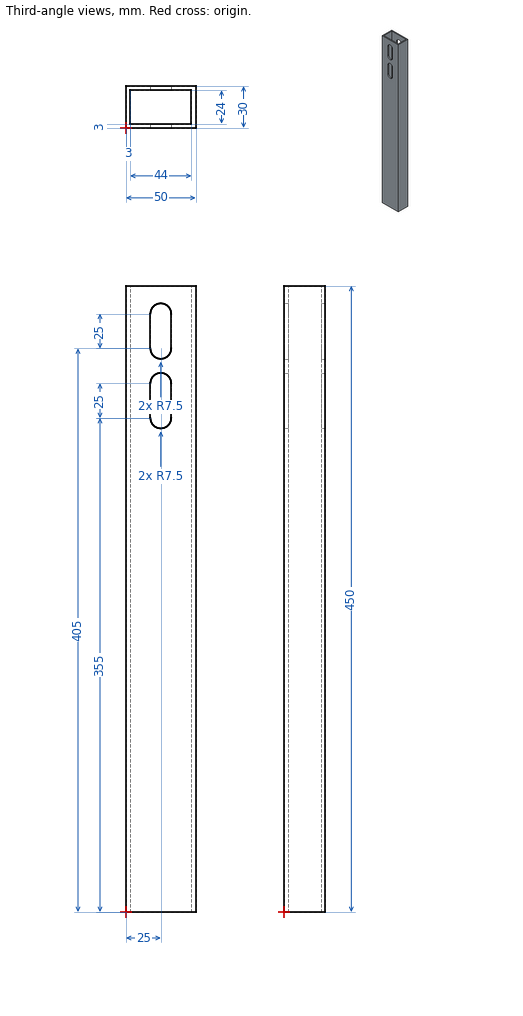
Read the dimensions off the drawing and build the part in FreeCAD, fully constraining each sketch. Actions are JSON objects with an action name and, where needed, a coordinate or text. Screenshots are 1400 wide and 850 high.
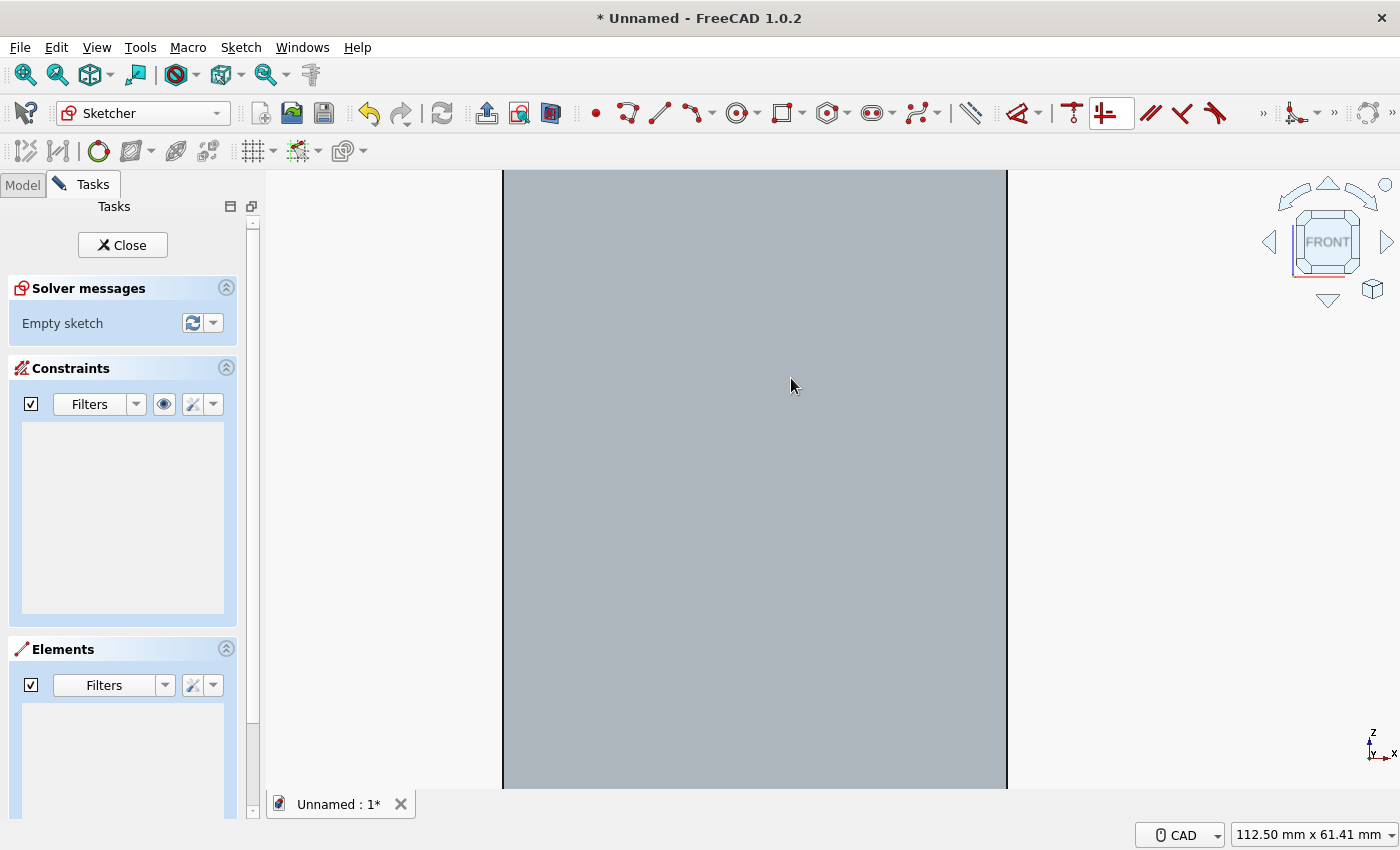
{"action": "left_click", "coordinate": [755, 609]}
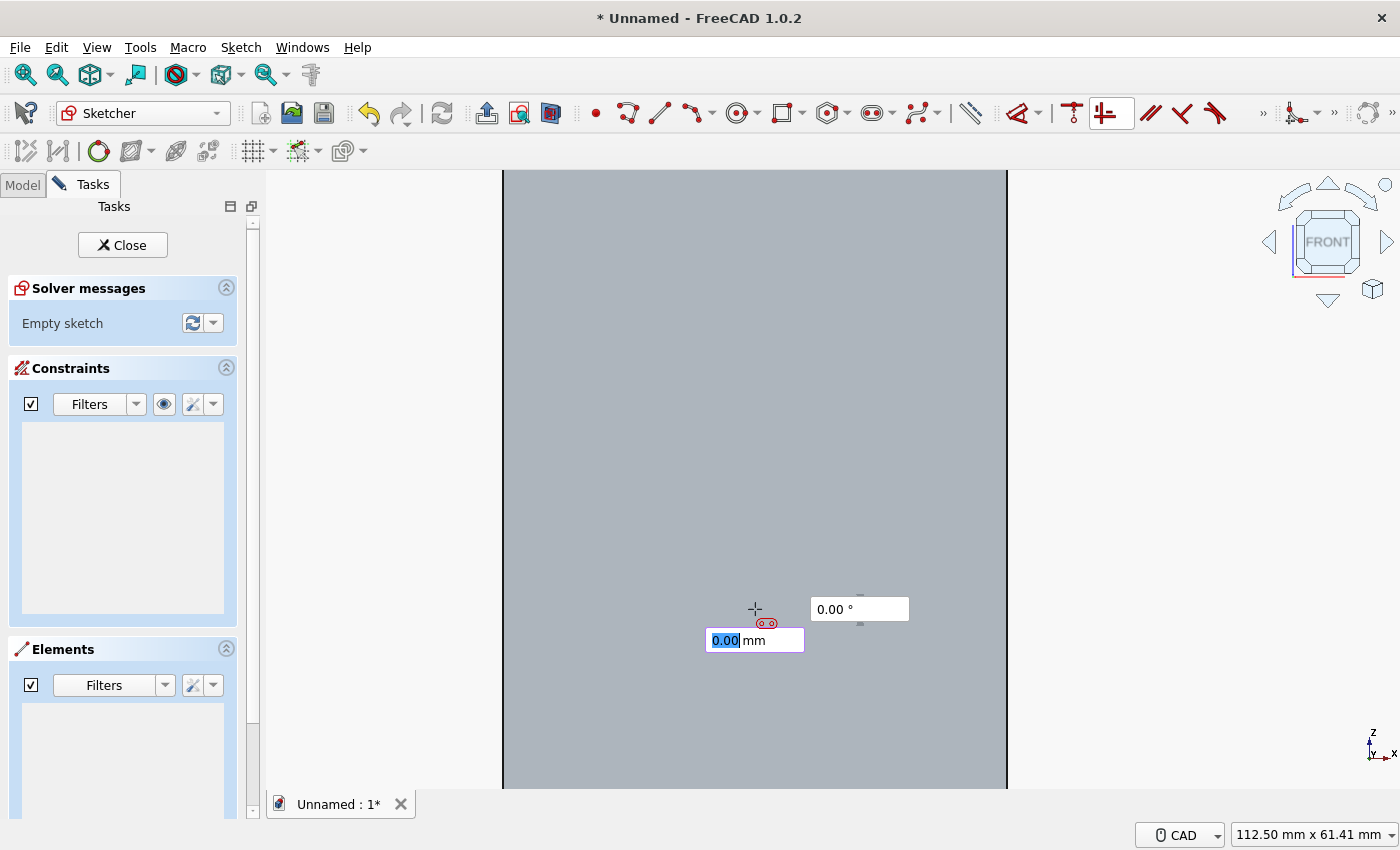
{"action": "left_click", "coordinate": [755, 357]}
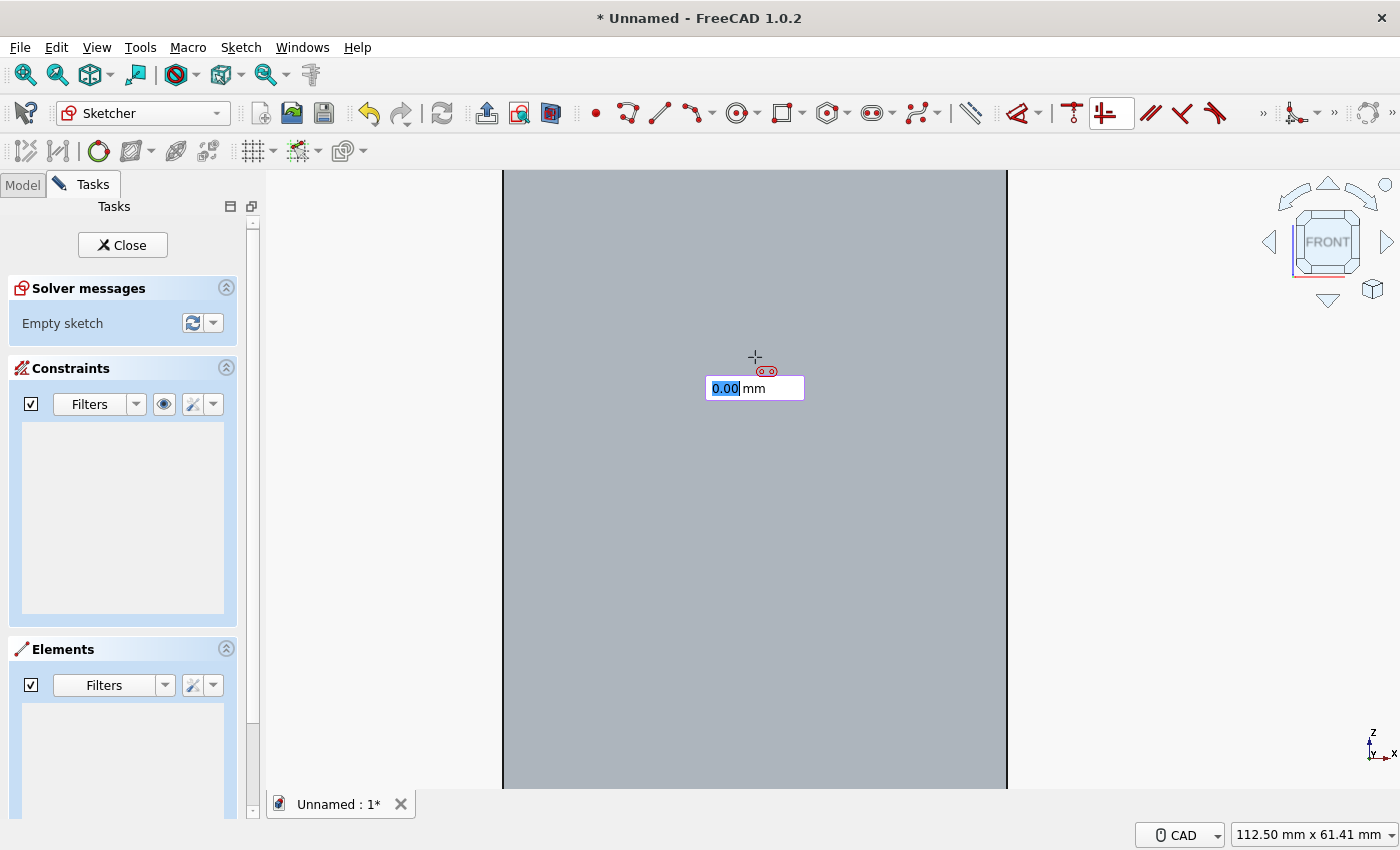
{"action": "left_click", "coordinate": [680, 483]}
{"action": "key", "text": "Escape"}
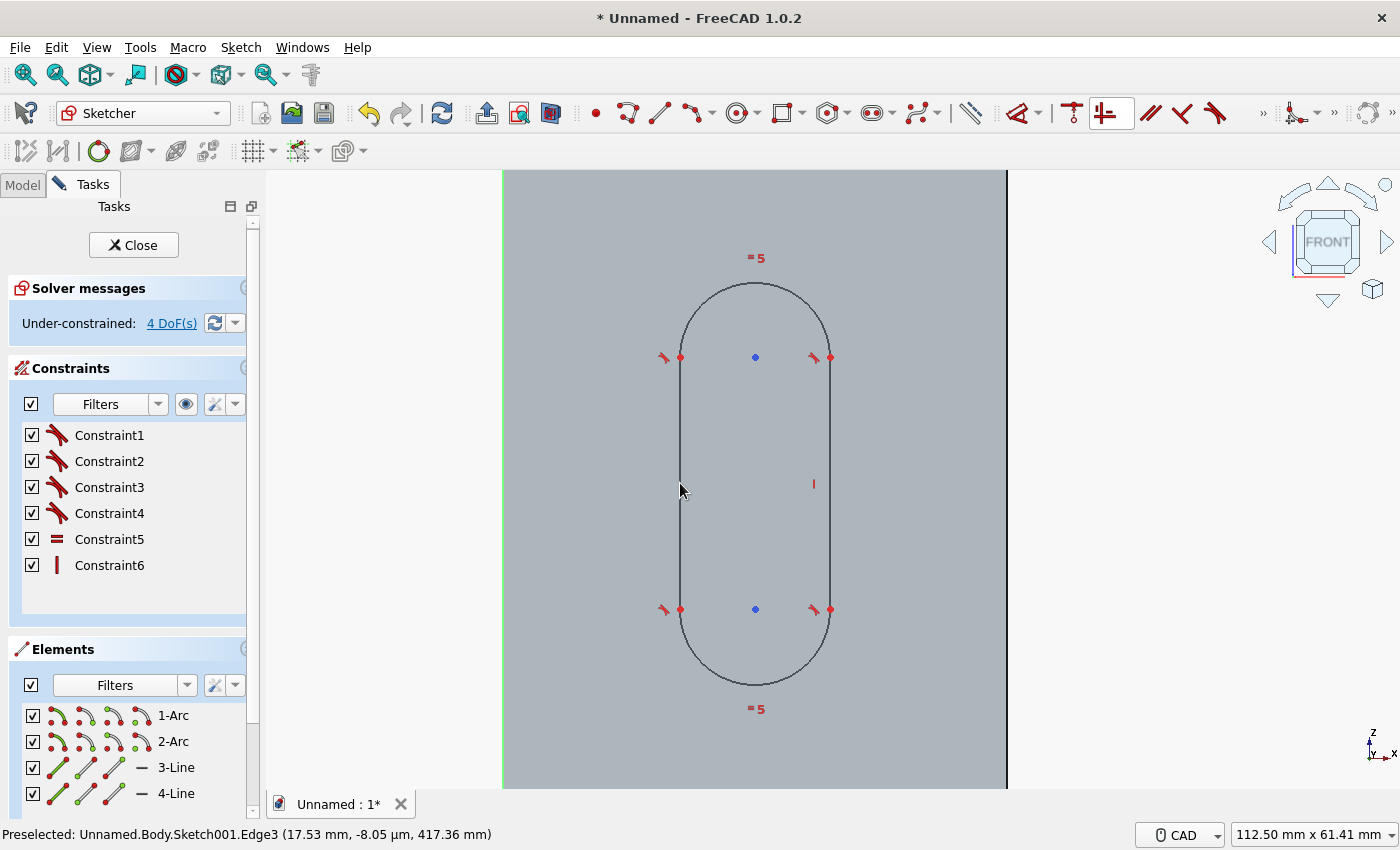
{"action": "left_click", "coordinate": [711, 671]}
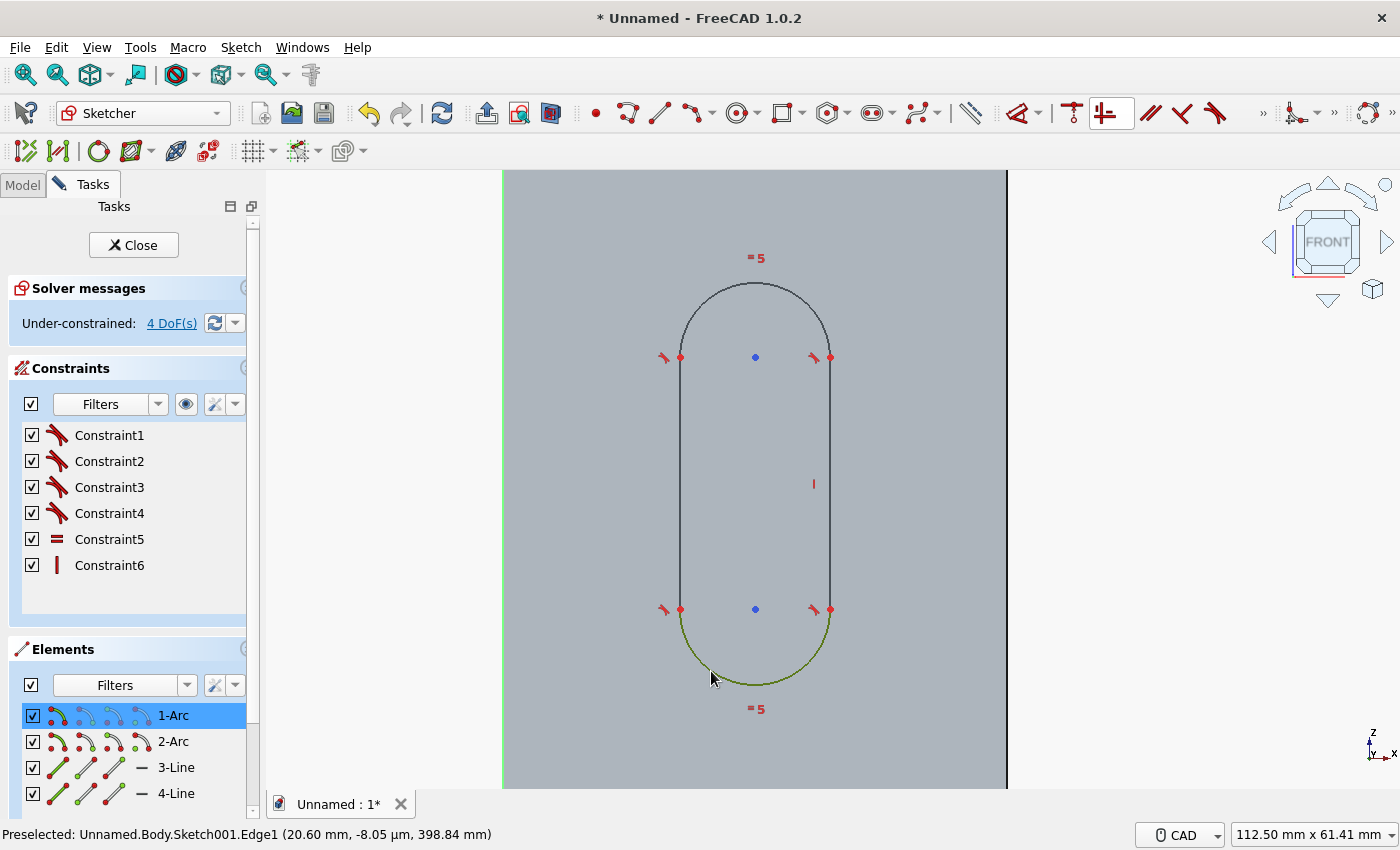
{"action": "key", "text": "k r"}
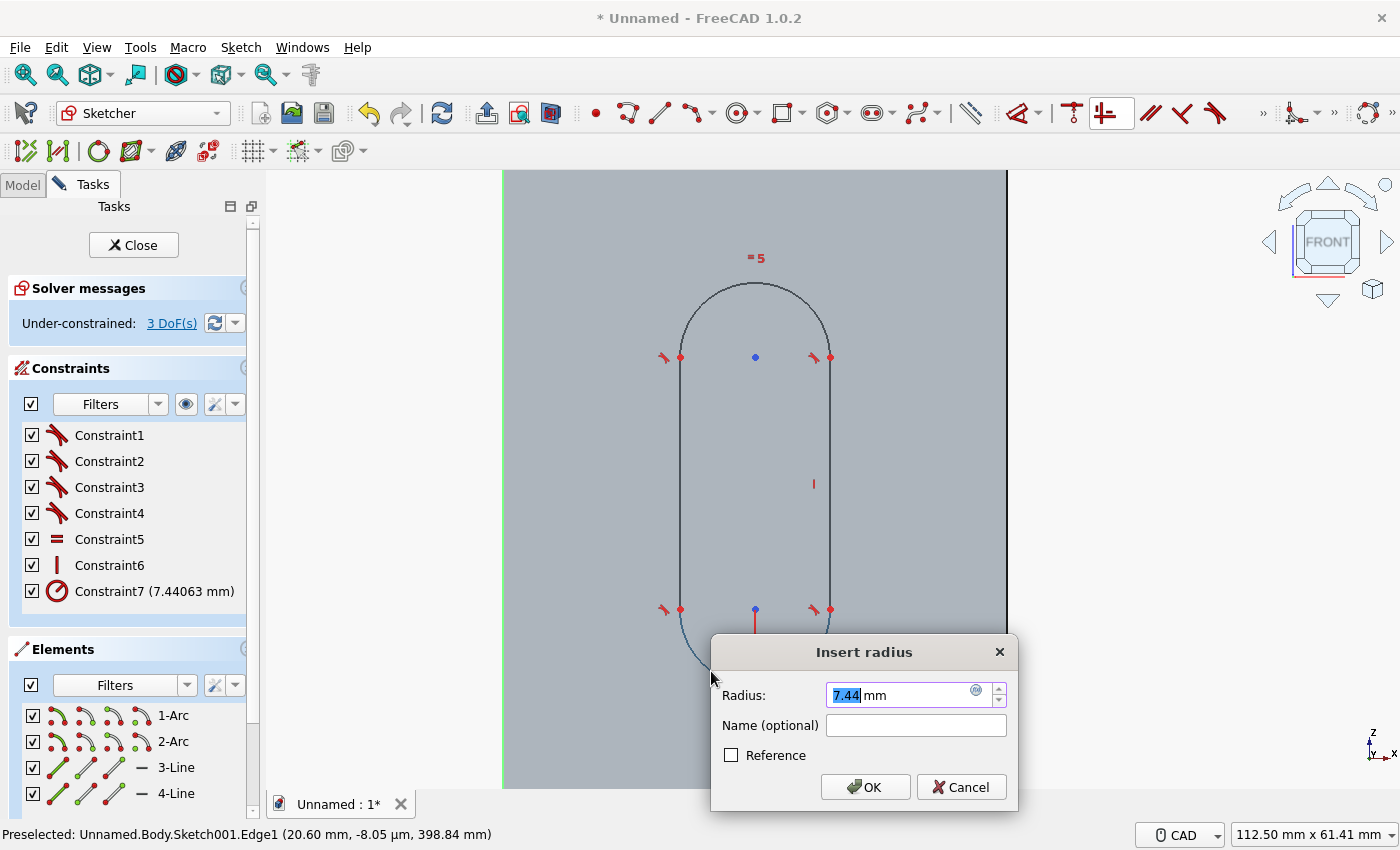
{"action": "type", "text": "7.5"}
{"action": "key", "text": "Return"}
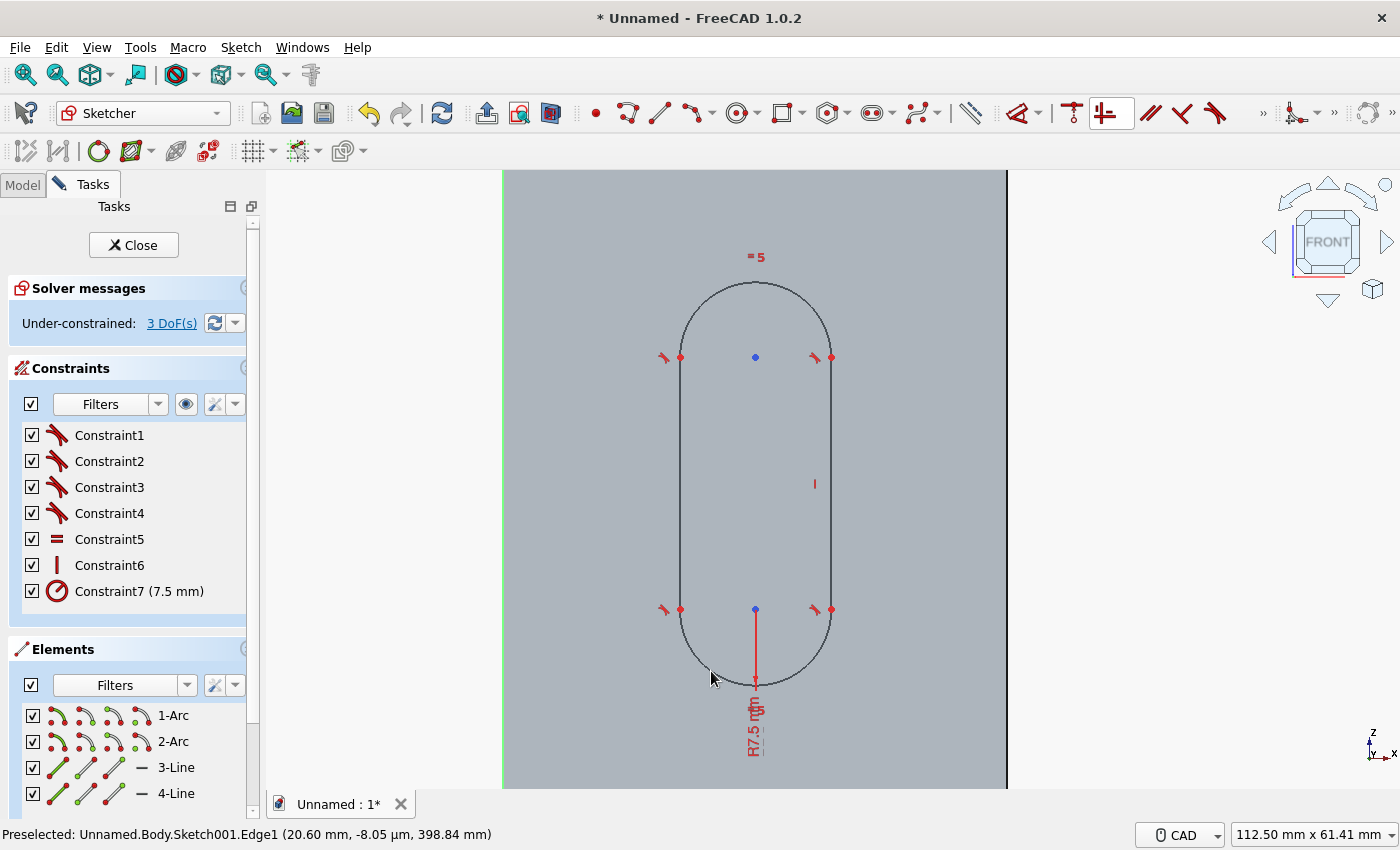
{"action": "left_click", "coordinate": [680, 534]}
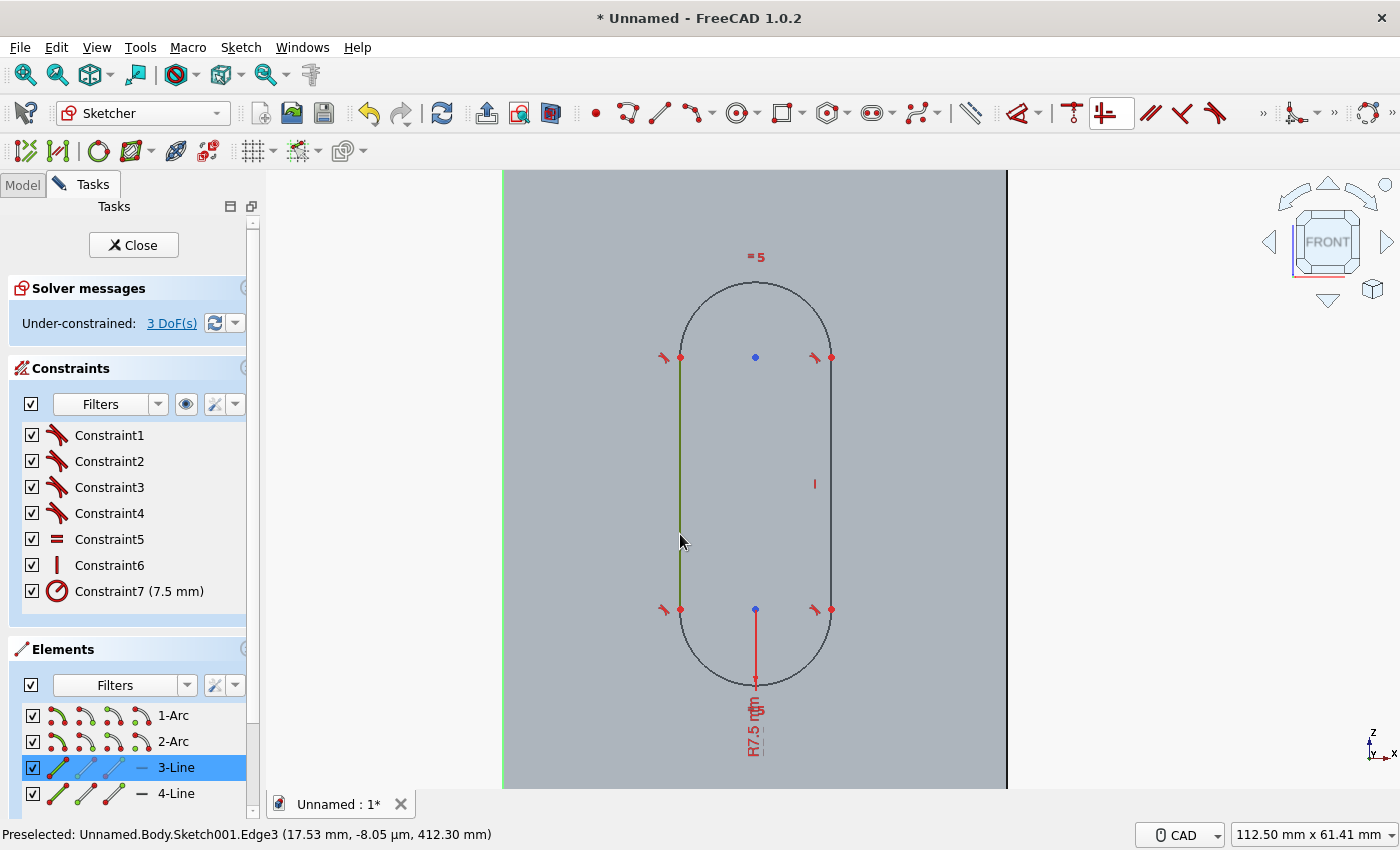
{"action": "key", "text": "i"}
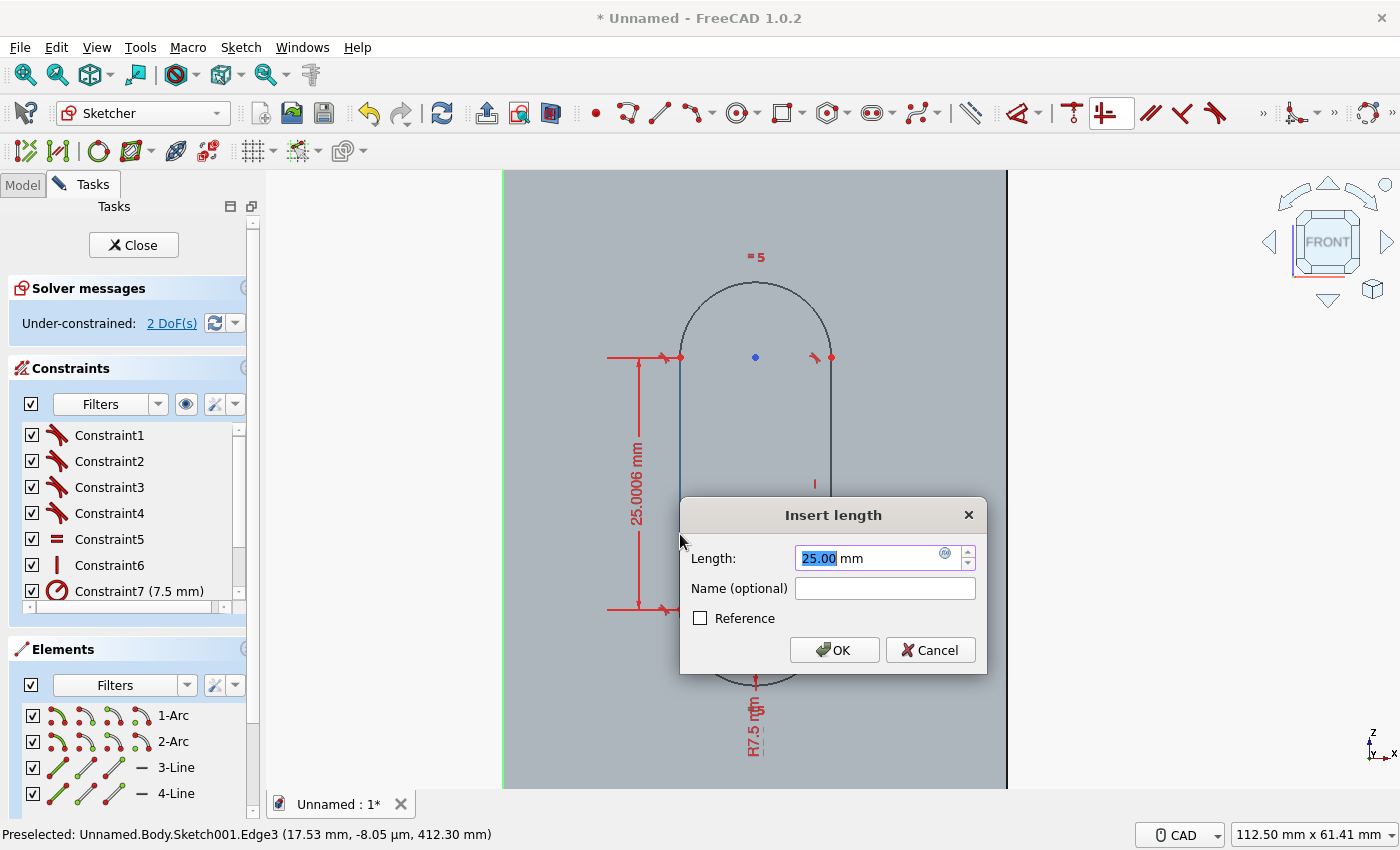
{"action": "type", "text": "25"}
{"action": "key", "text": "Return"}